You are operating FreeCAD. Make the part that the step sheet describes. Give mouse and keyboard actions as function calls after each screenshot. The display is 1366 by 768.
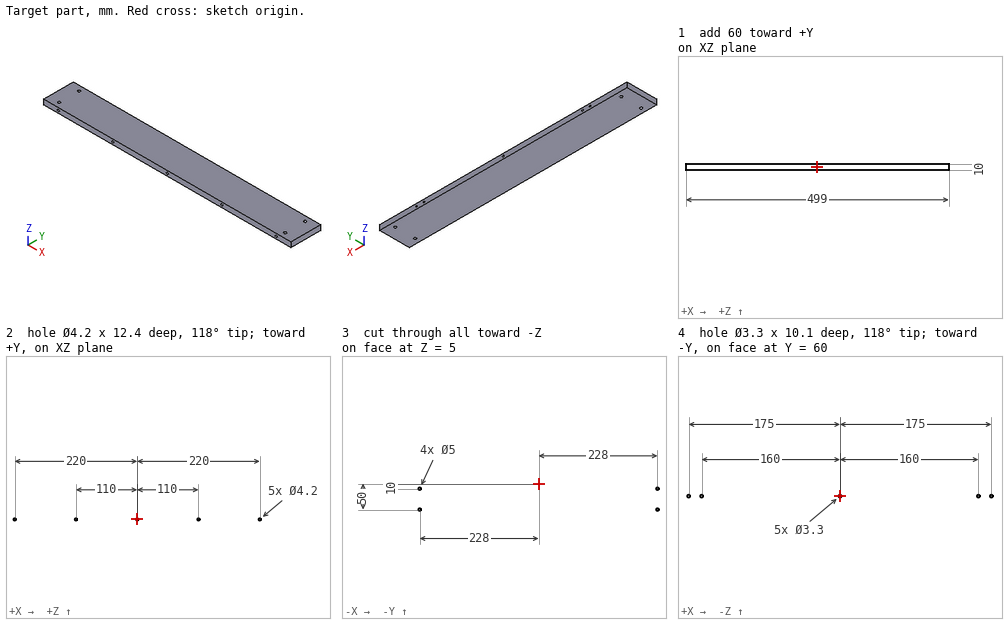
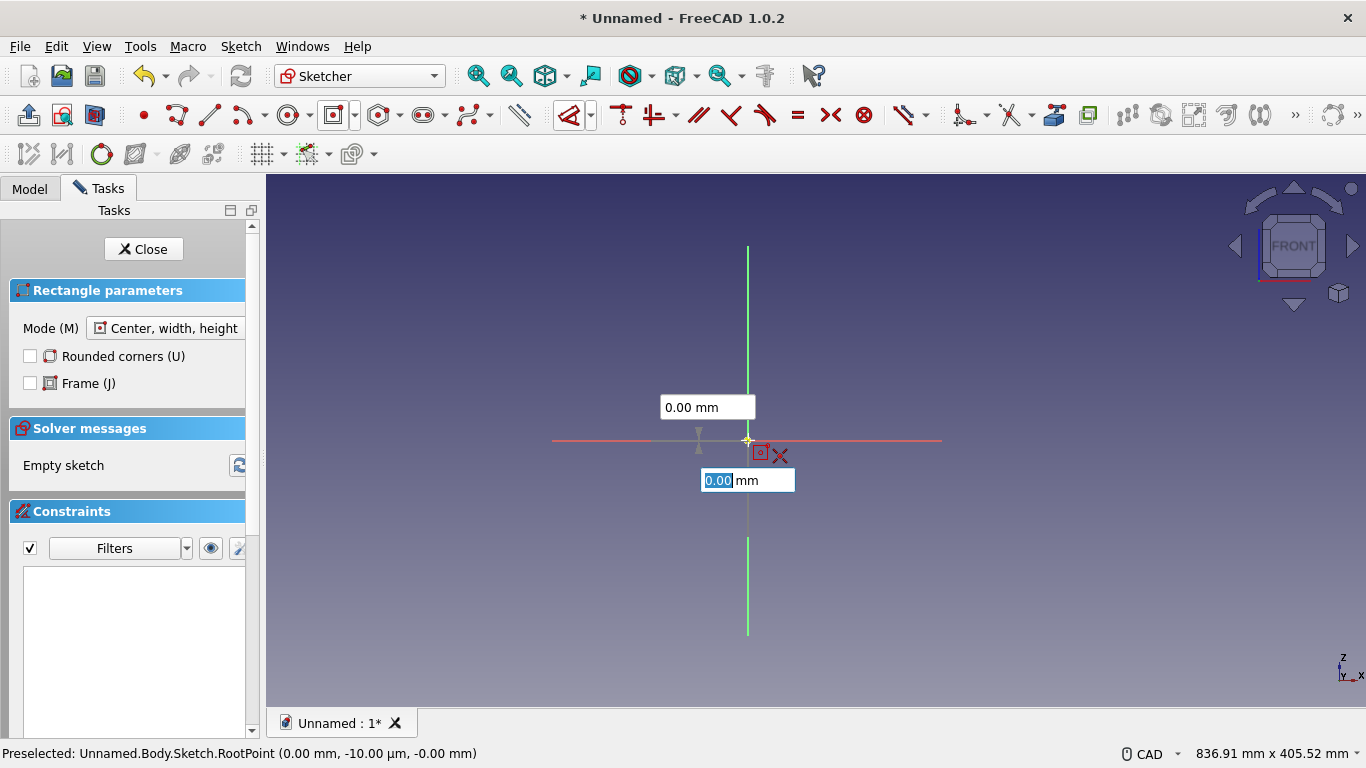
scroll(1076, 434, up, 5)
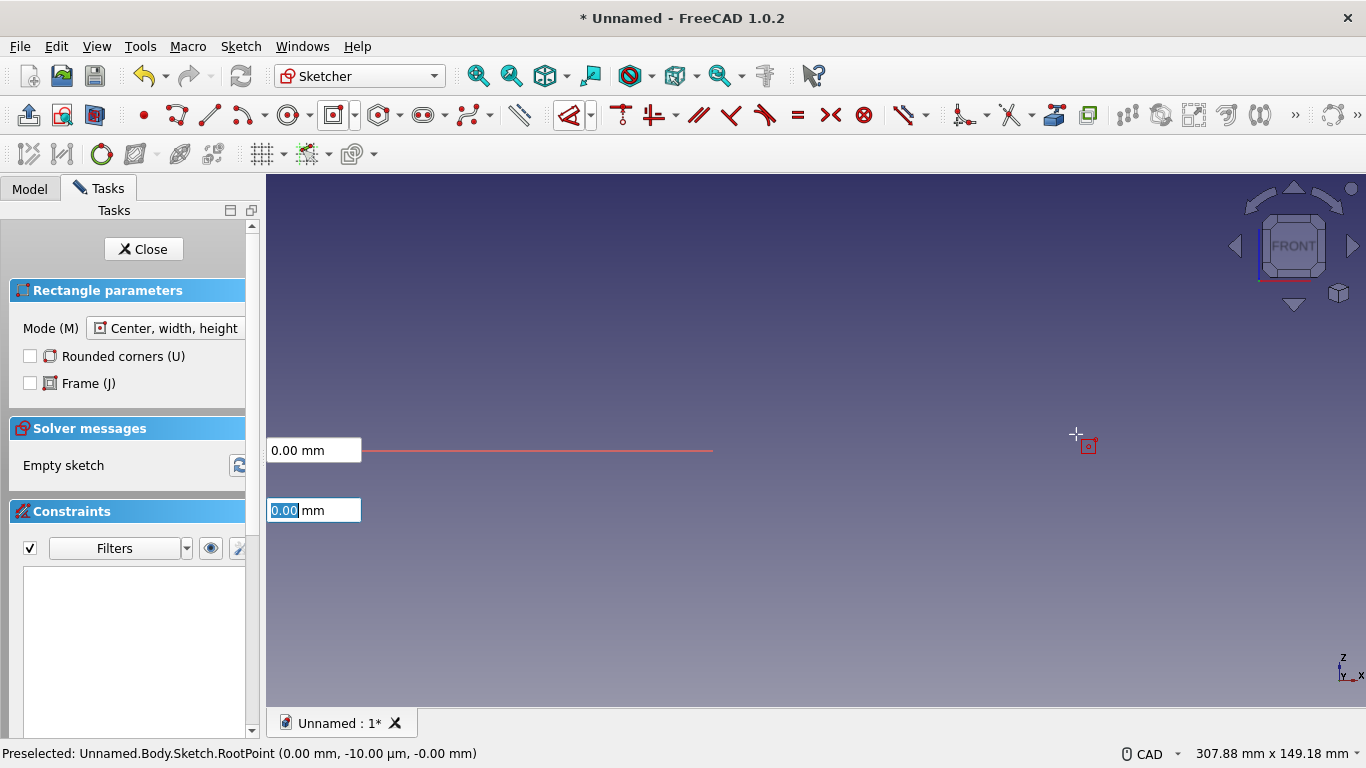
click(1074, 433)
key(Escape)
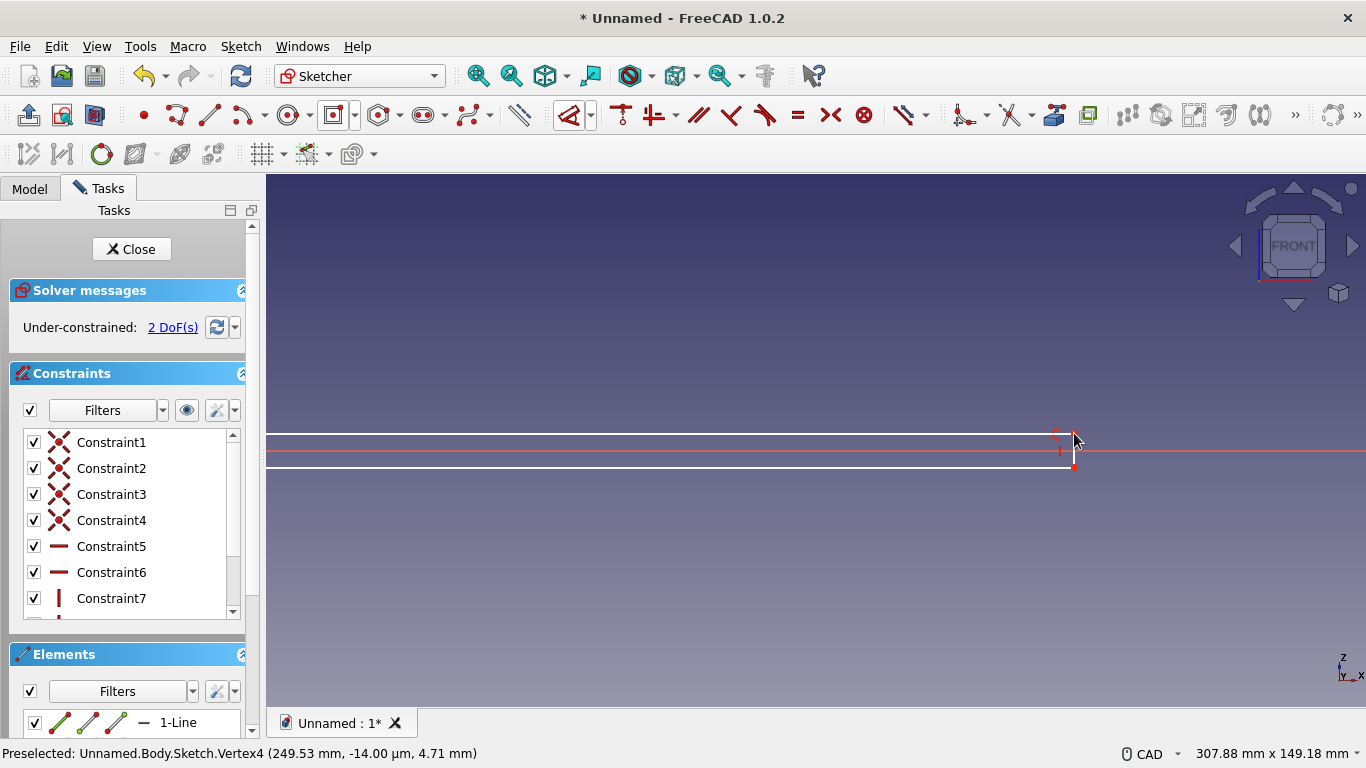
key(d)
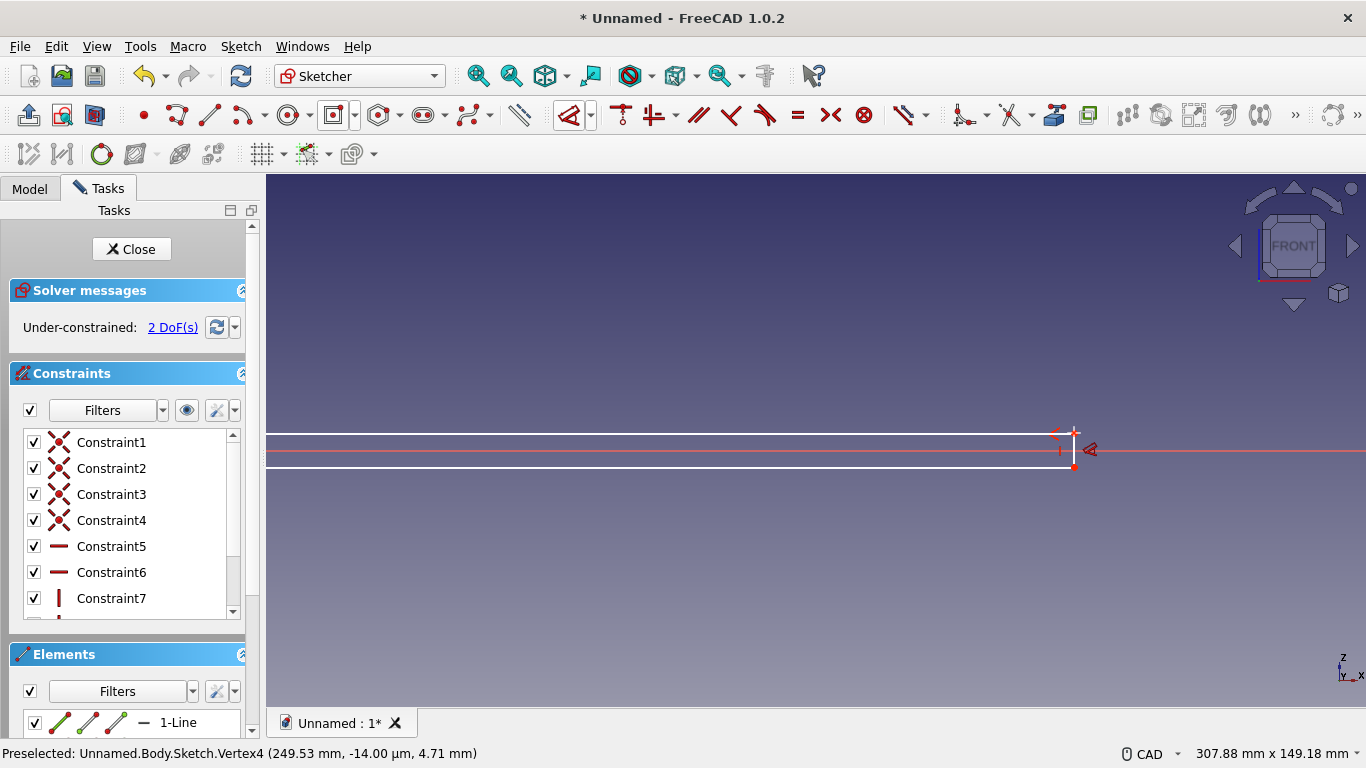
click(1074, 454)
click(1108, 443)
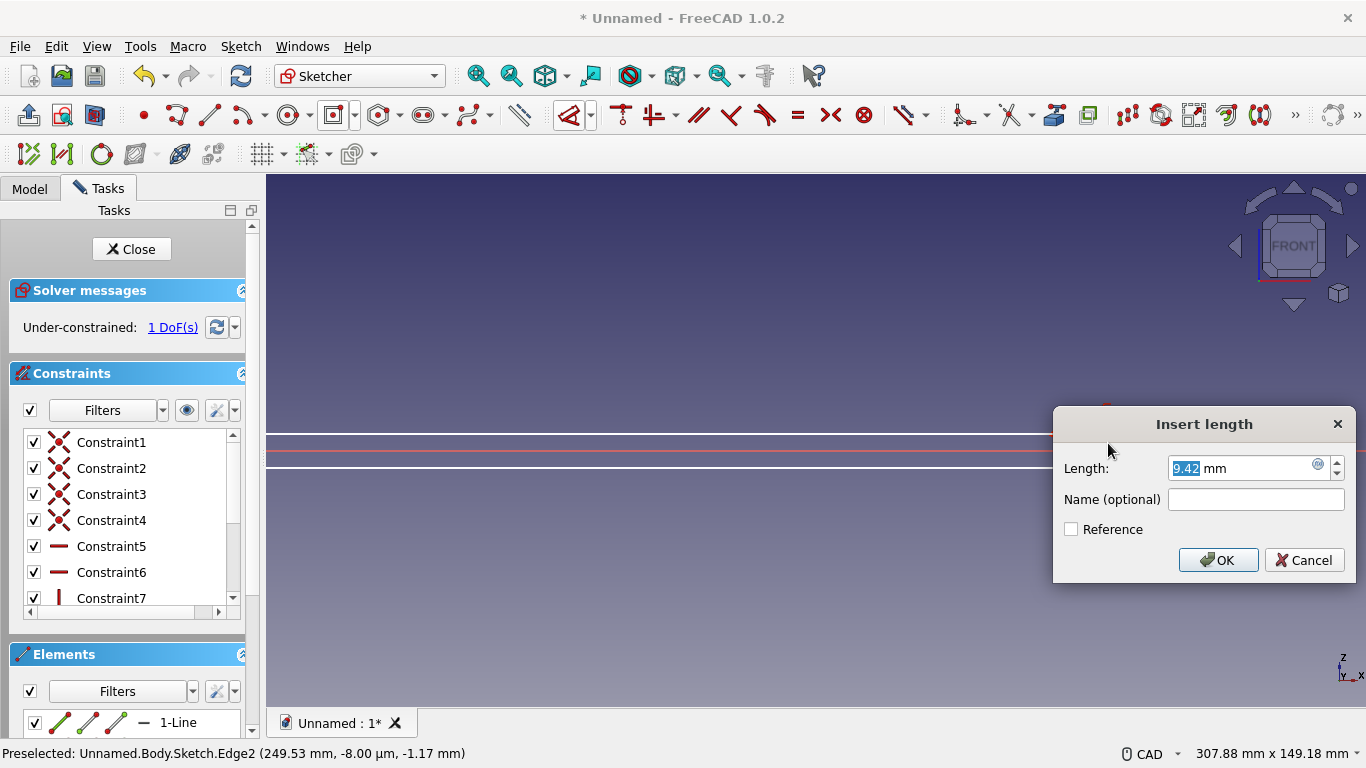
text(10)
key(Return)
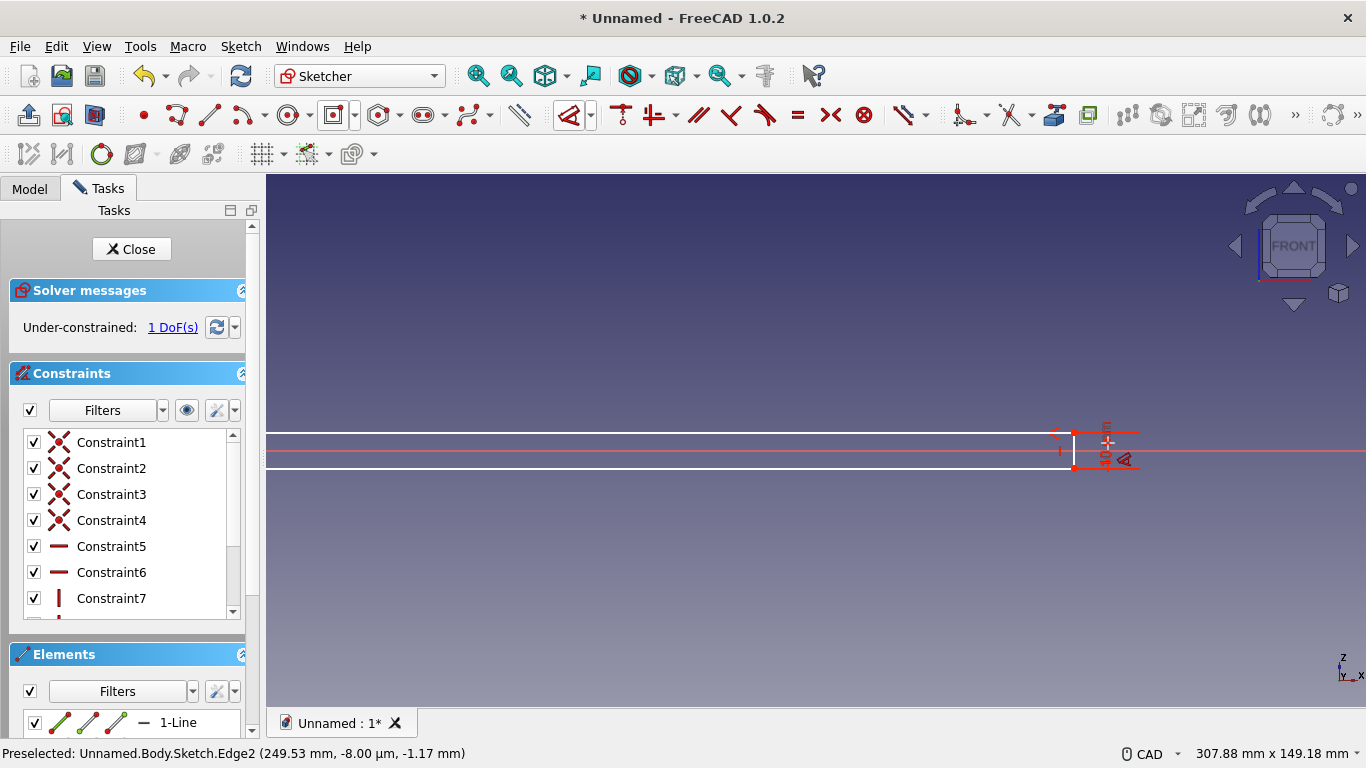
click(539, 469)
click(684, 503)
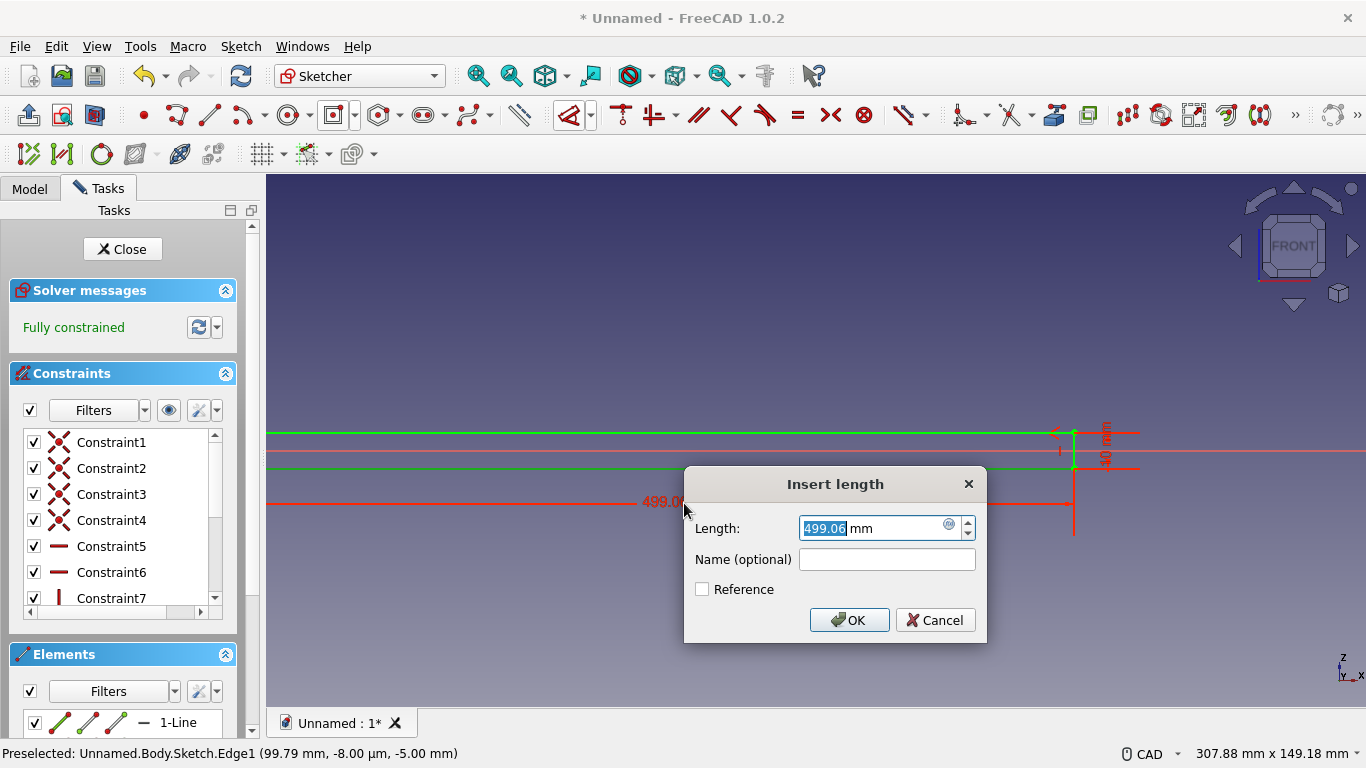
text(499)
key(Return)
key(Escape)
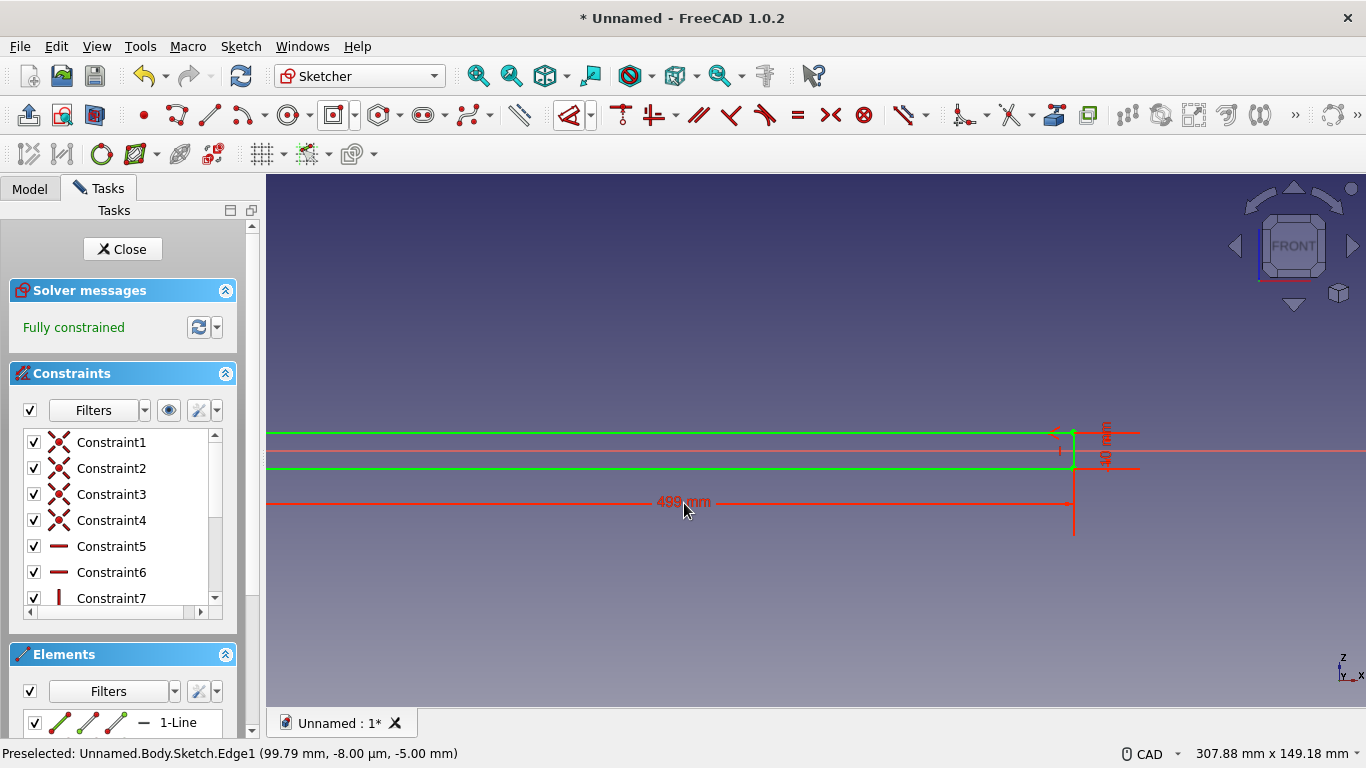
click(123, 249)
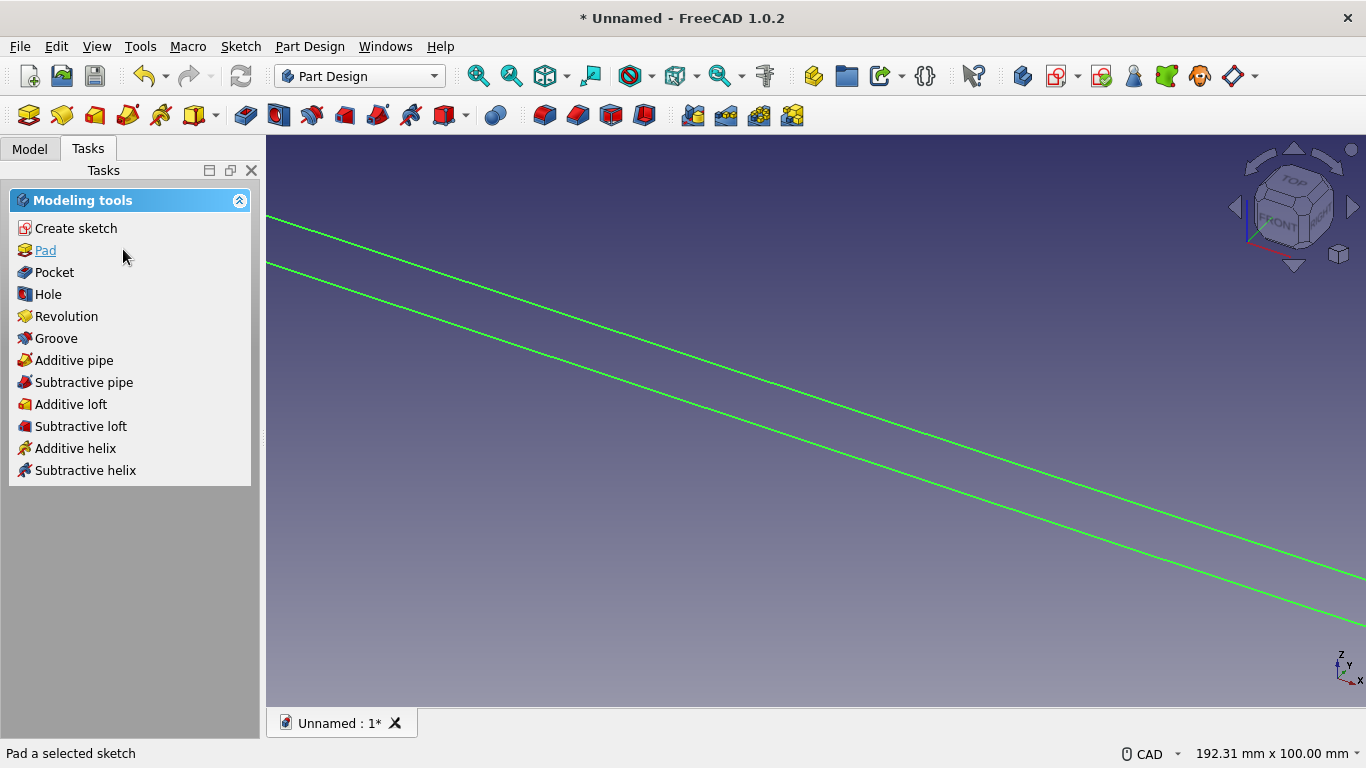
click(29, 116)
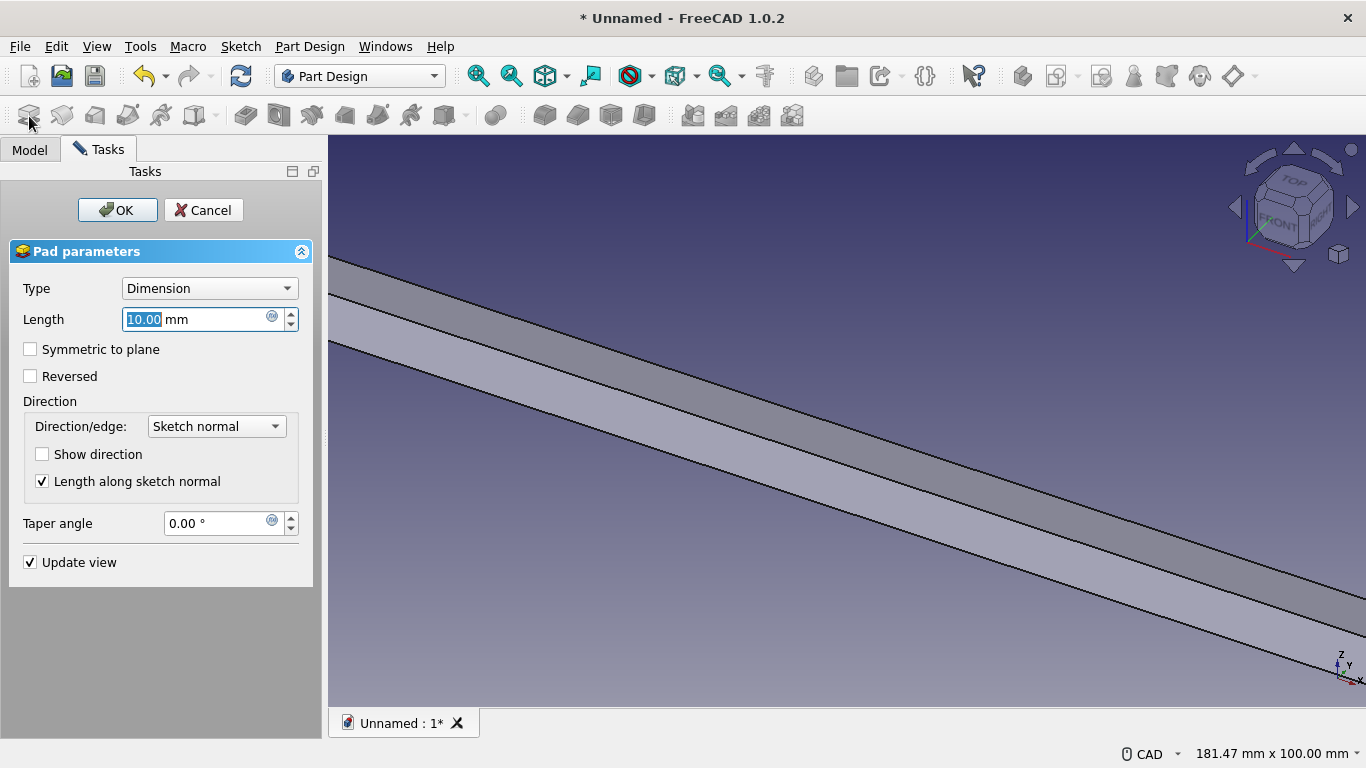
text(60)
key(Tab)